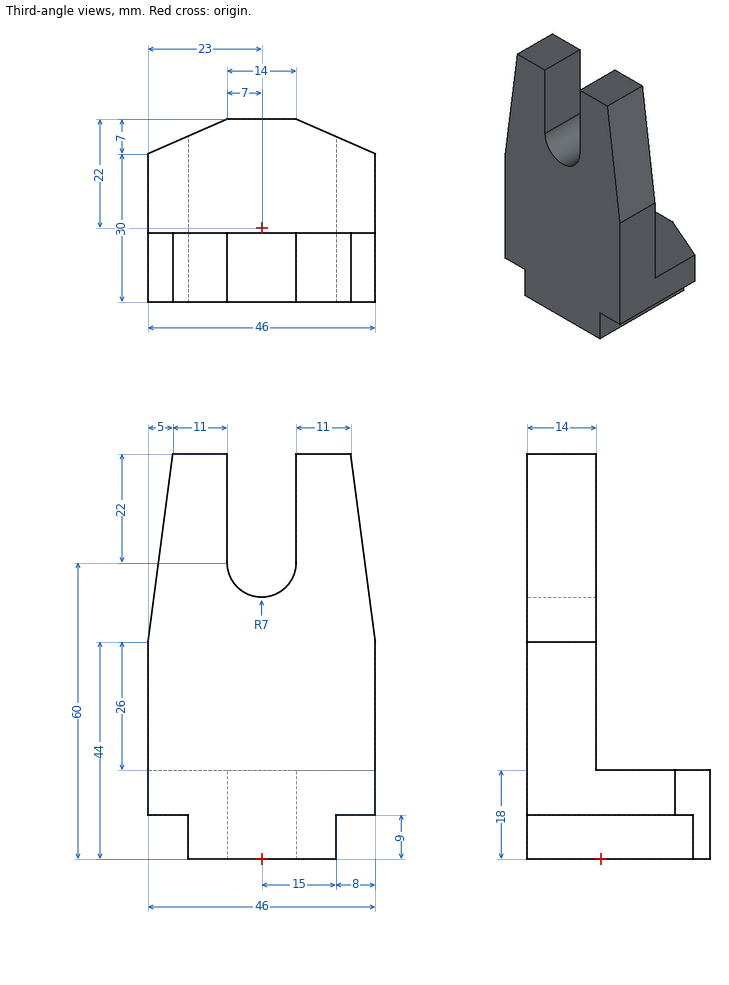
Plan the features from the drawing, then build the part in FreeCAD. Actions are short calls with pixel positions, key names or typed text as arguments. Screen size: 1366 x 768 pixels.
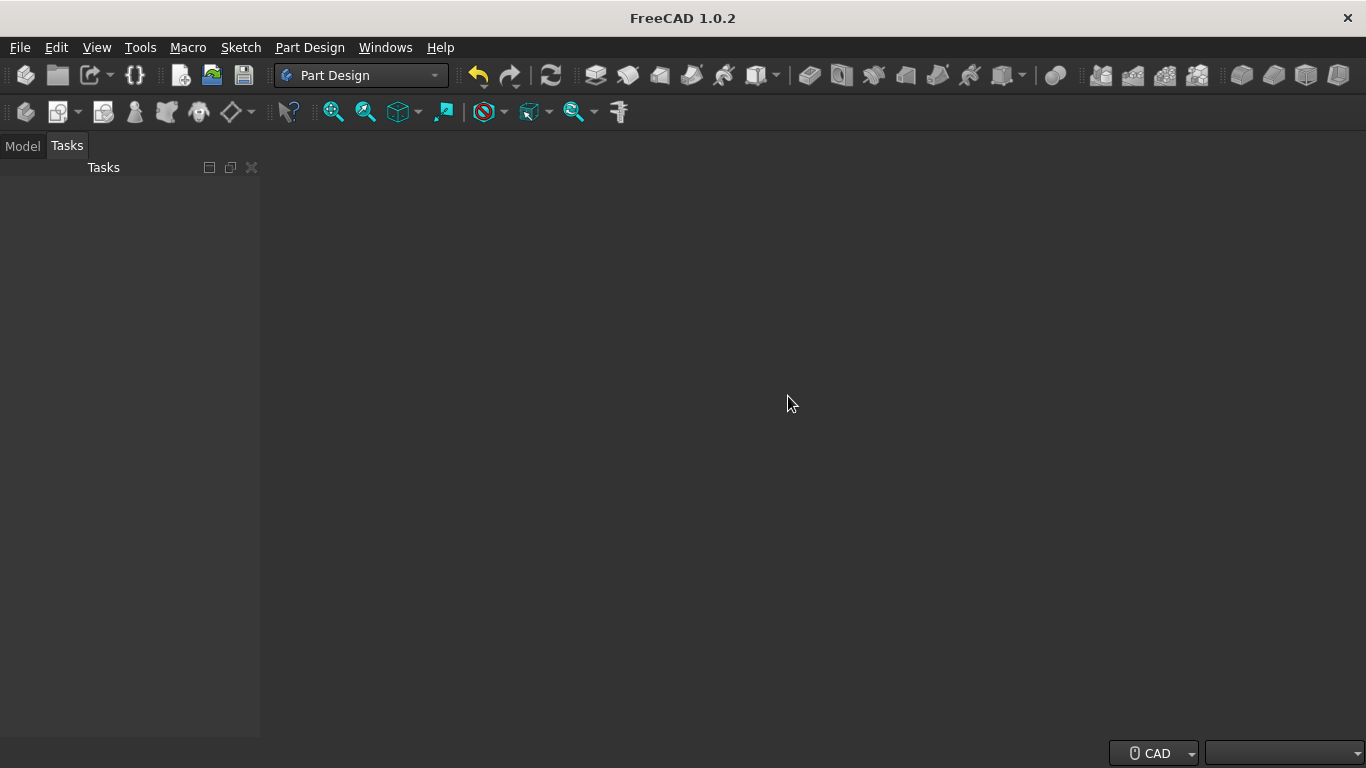
click(180, 76)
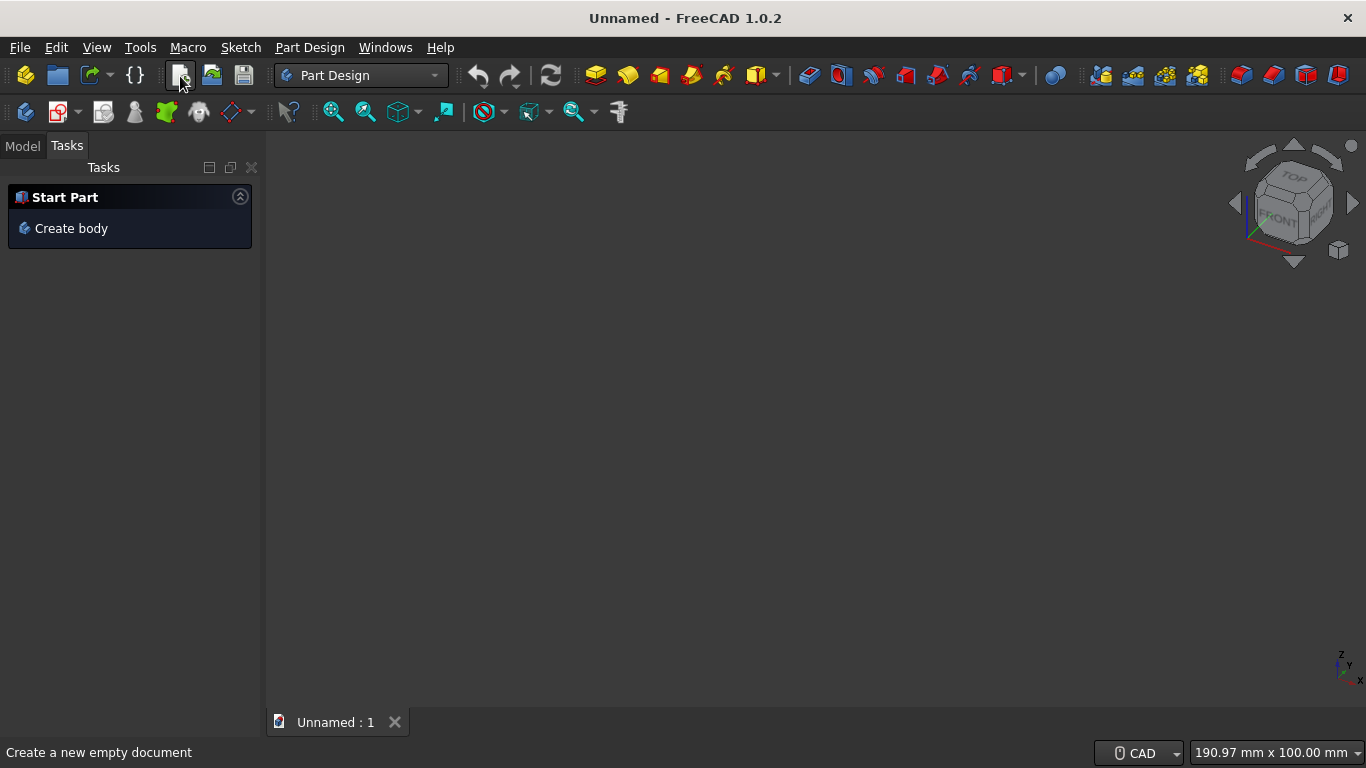
click(58, 112)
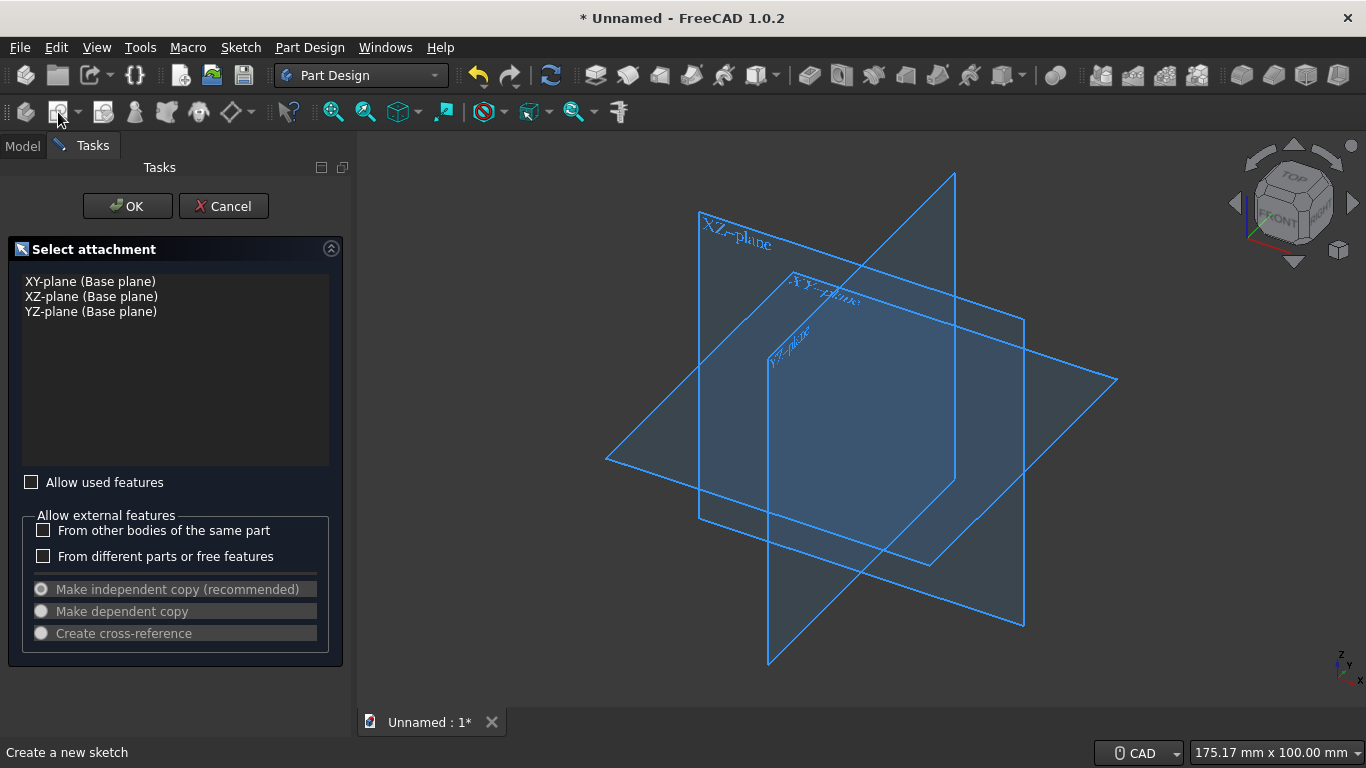
click(82, 282)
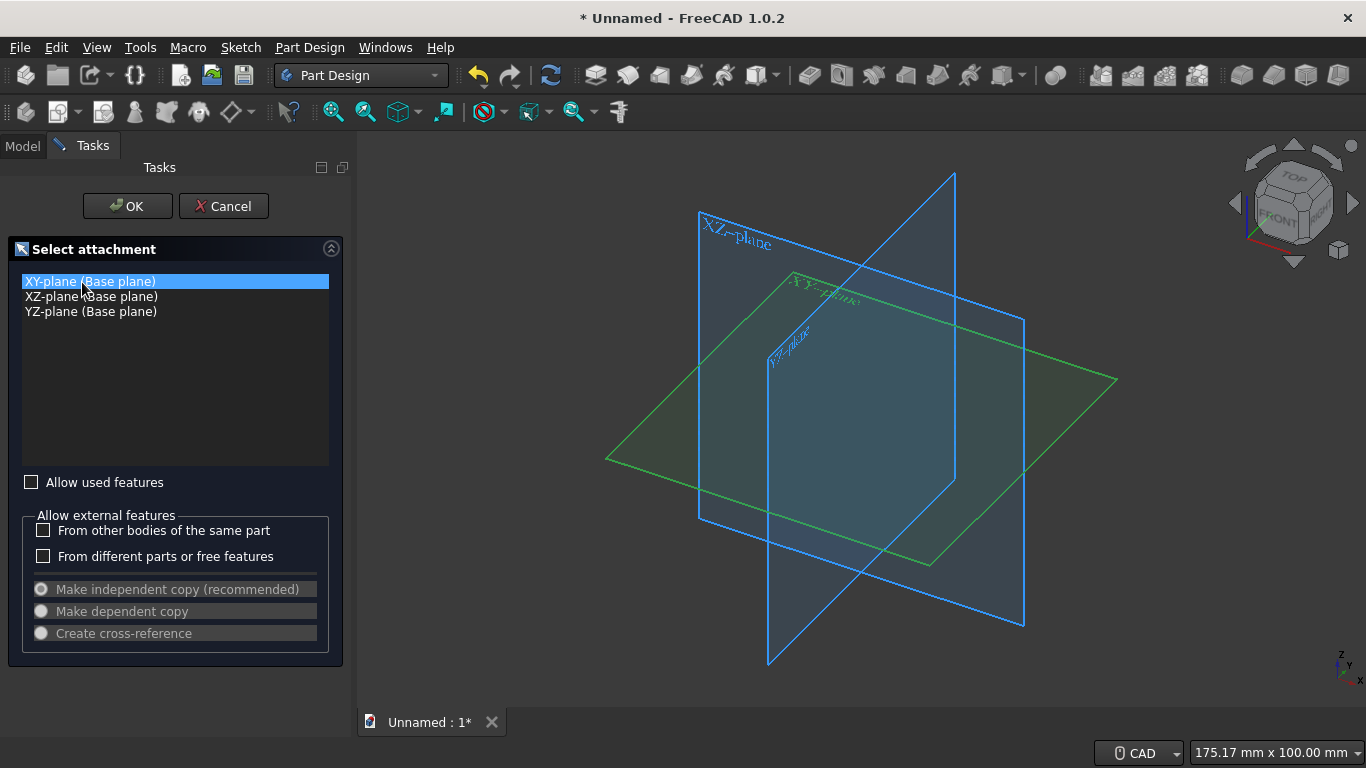
click(128, 206)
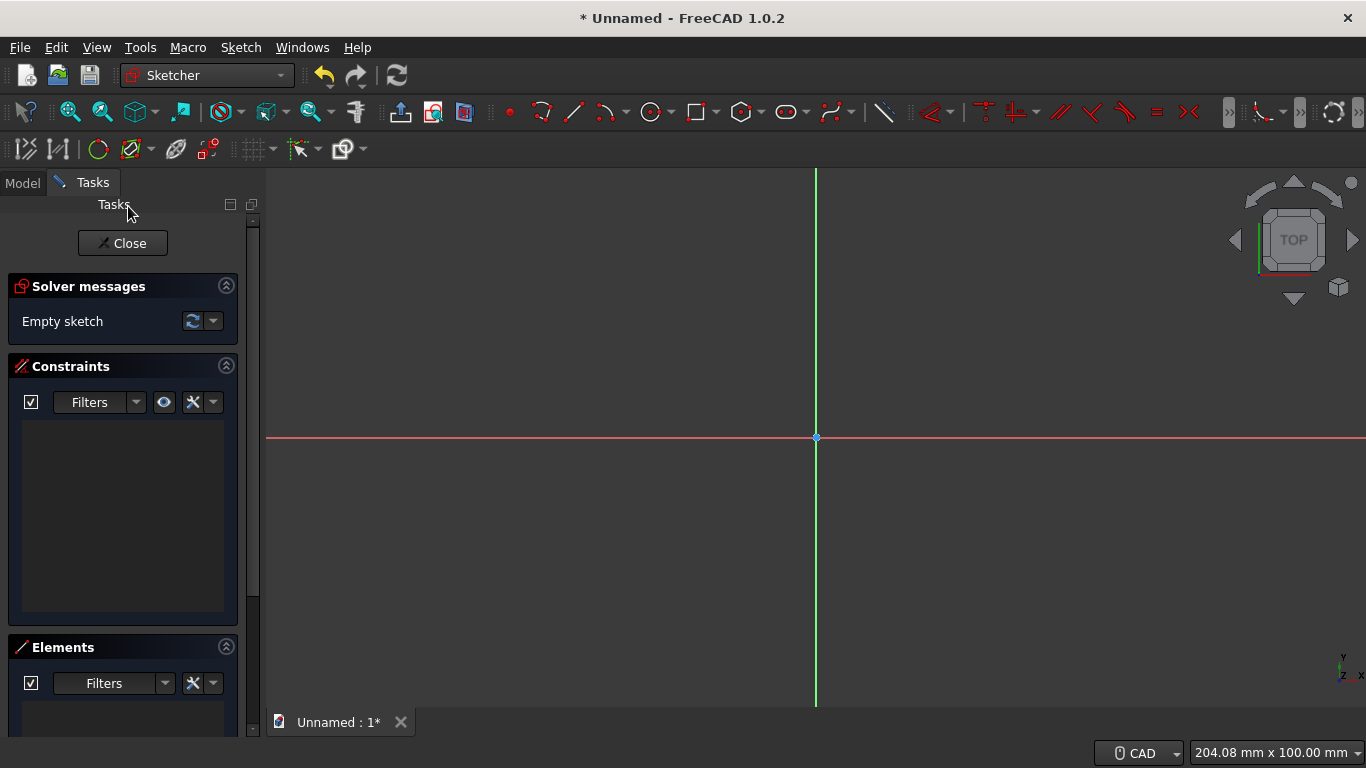
scroll(899, 396, up, 3)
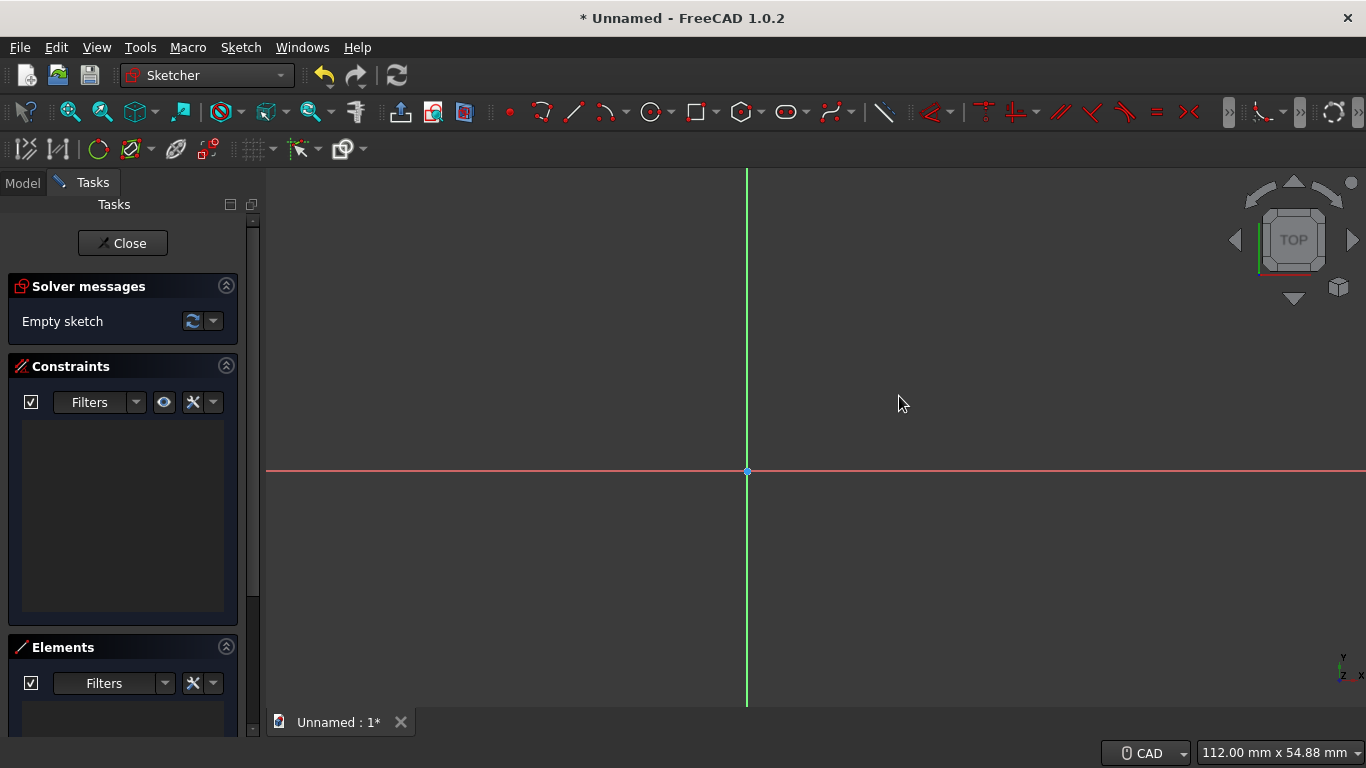
click(542, 112)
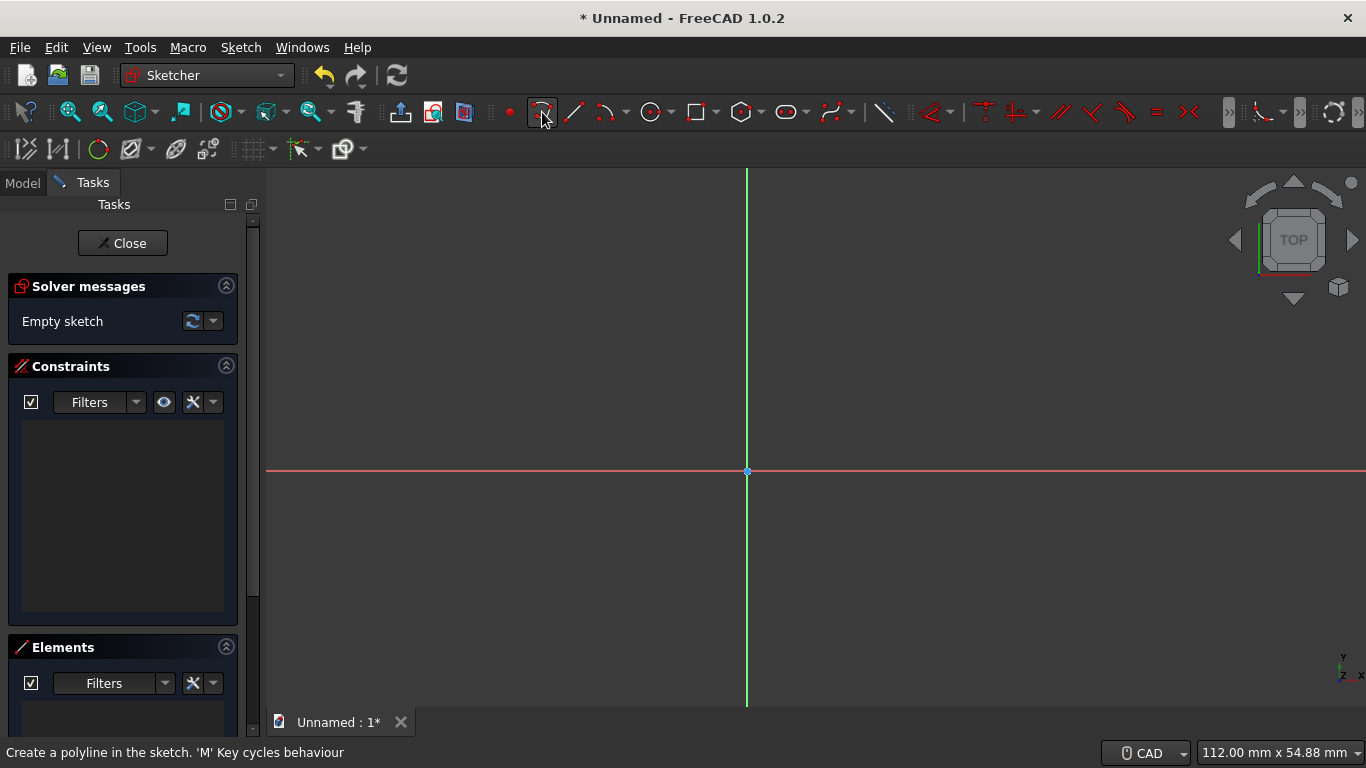
click(679, 255)
click(521, 324)
click(521, 619)
click(973, 619)
click(973, 324)
click(816, 255)
click(679, 256)
key(Escape)
key(Escape)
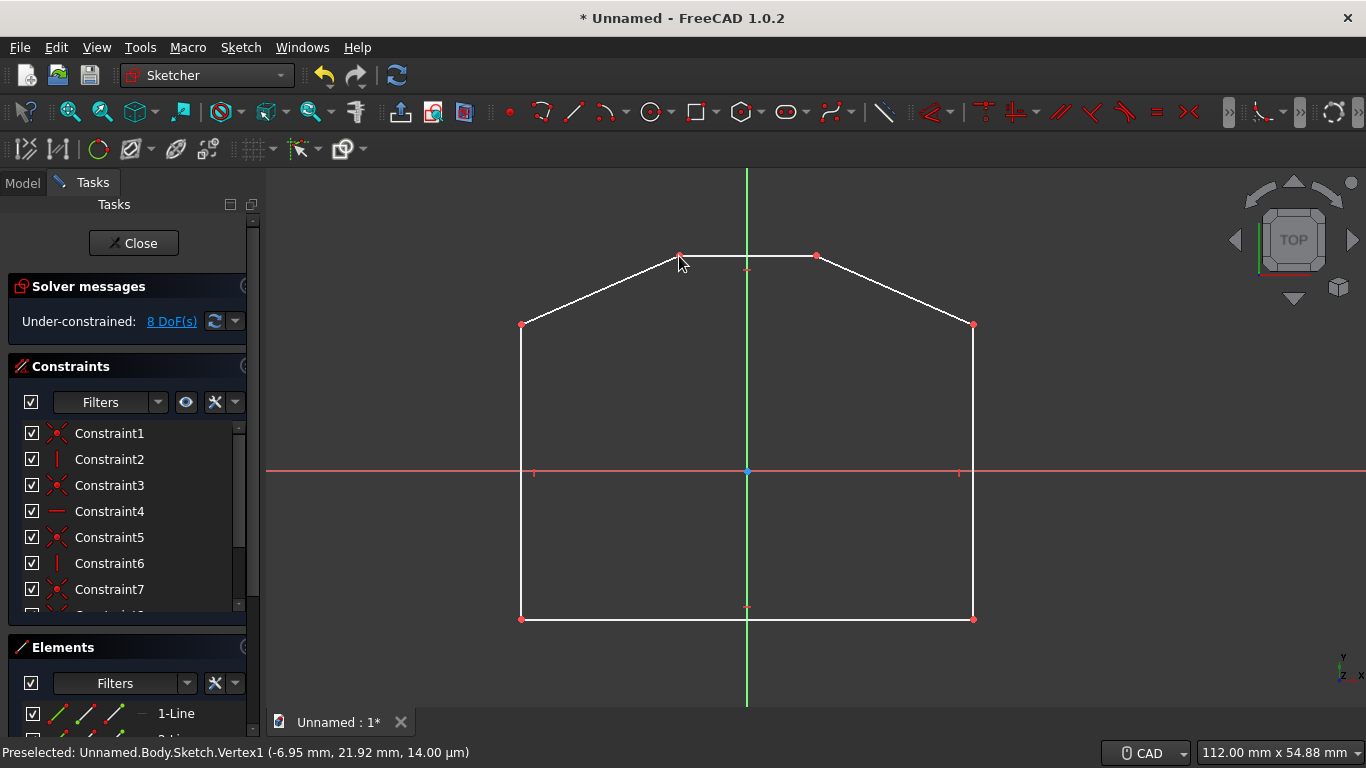
click(521, 414)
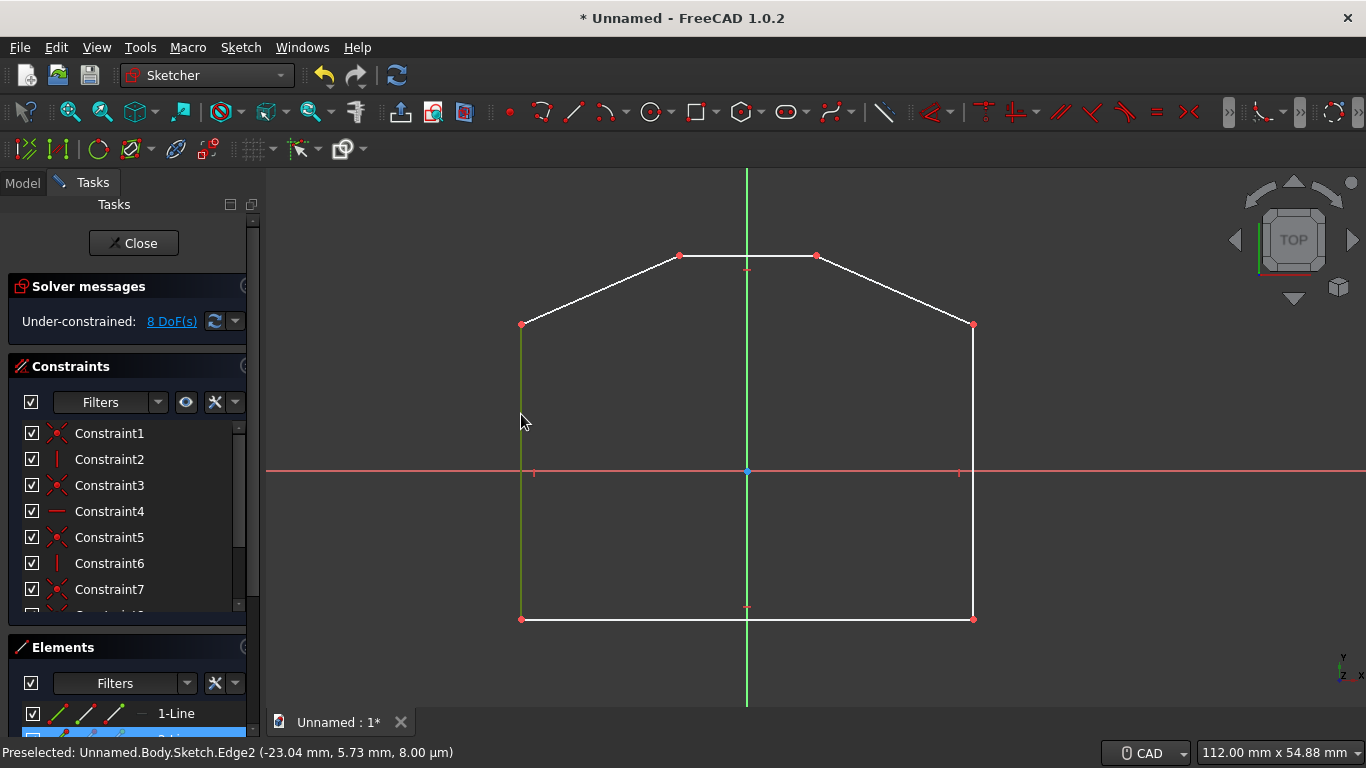
click(952, 112)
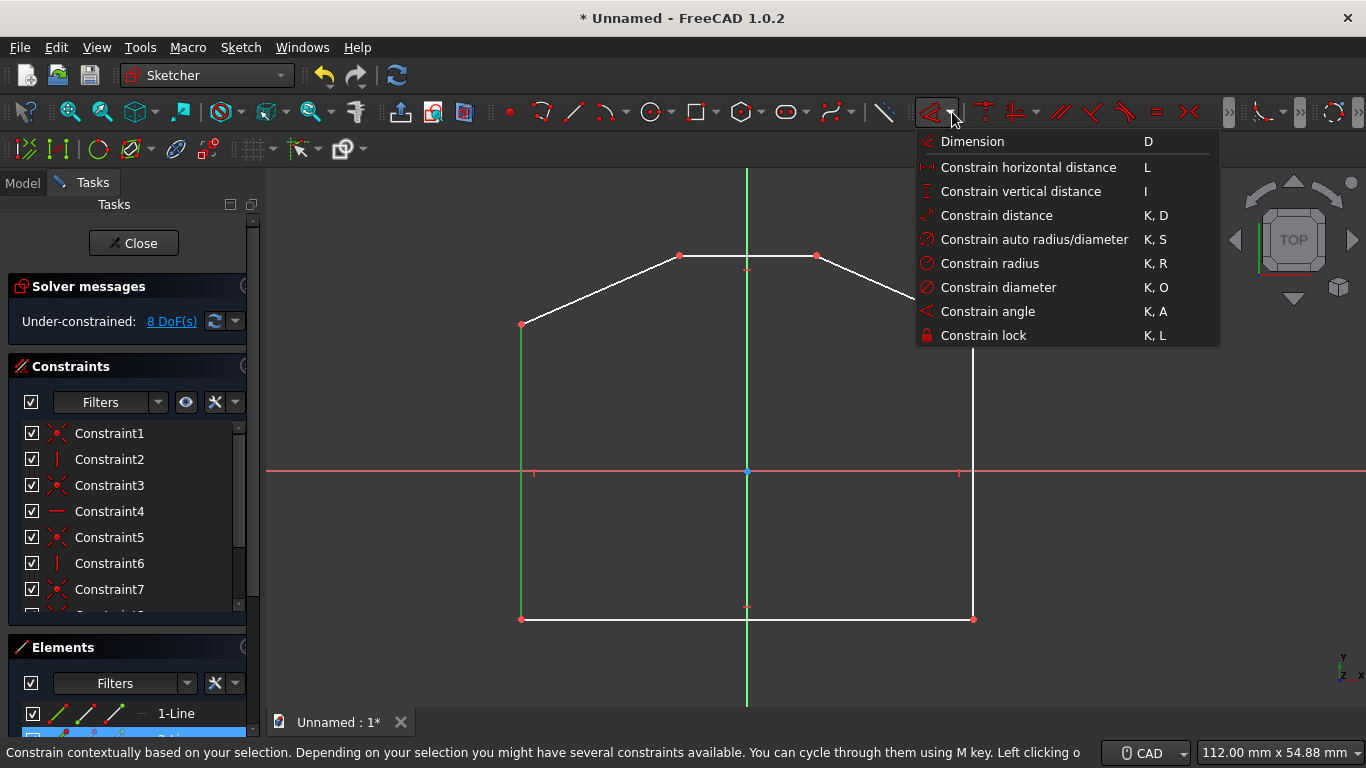
click(1068, 191)